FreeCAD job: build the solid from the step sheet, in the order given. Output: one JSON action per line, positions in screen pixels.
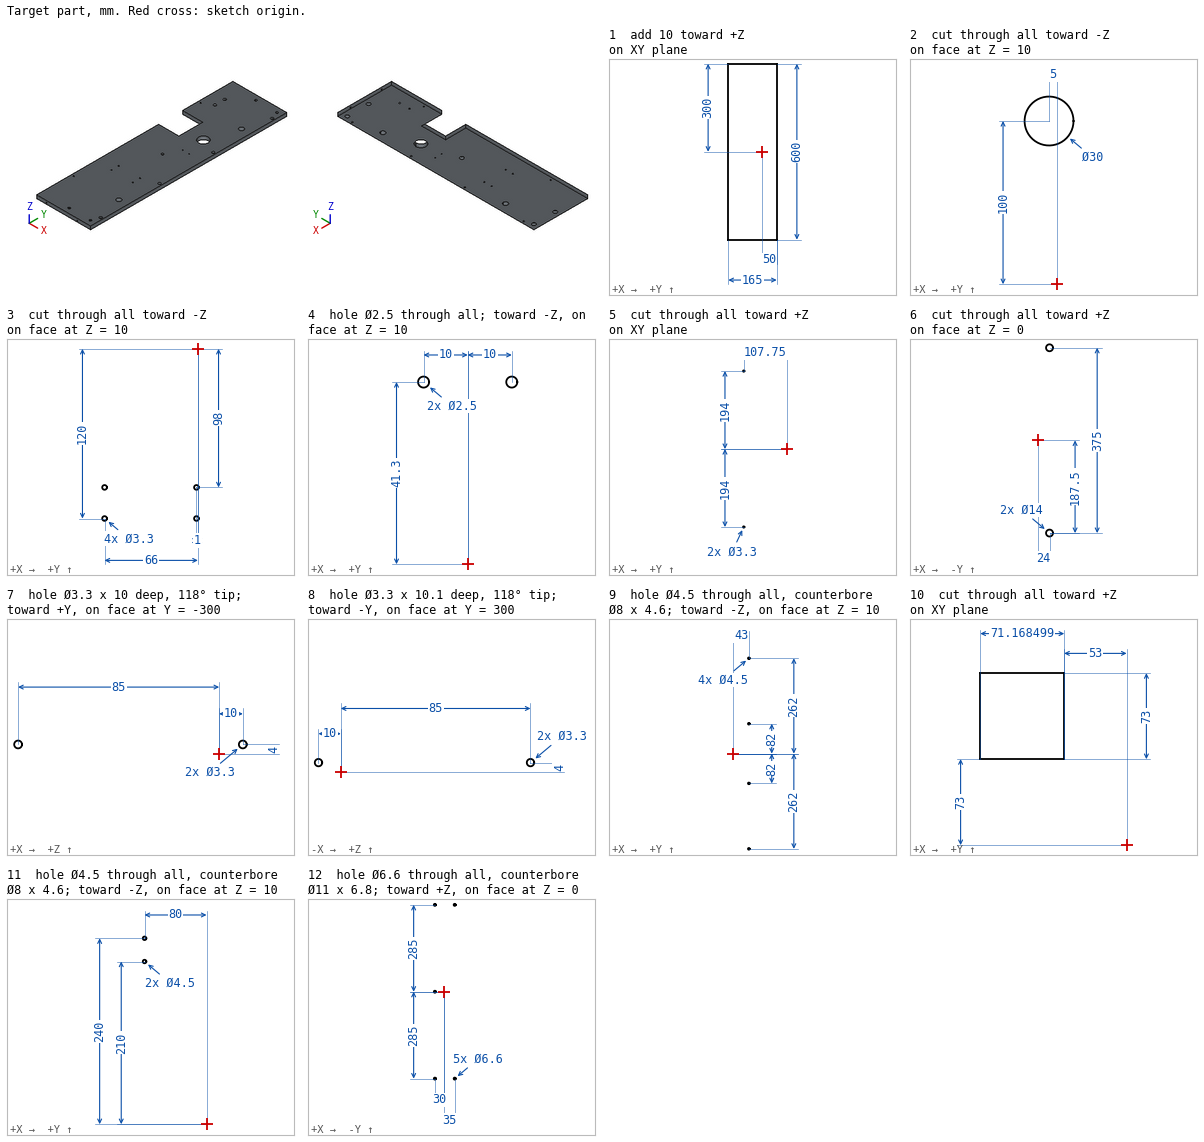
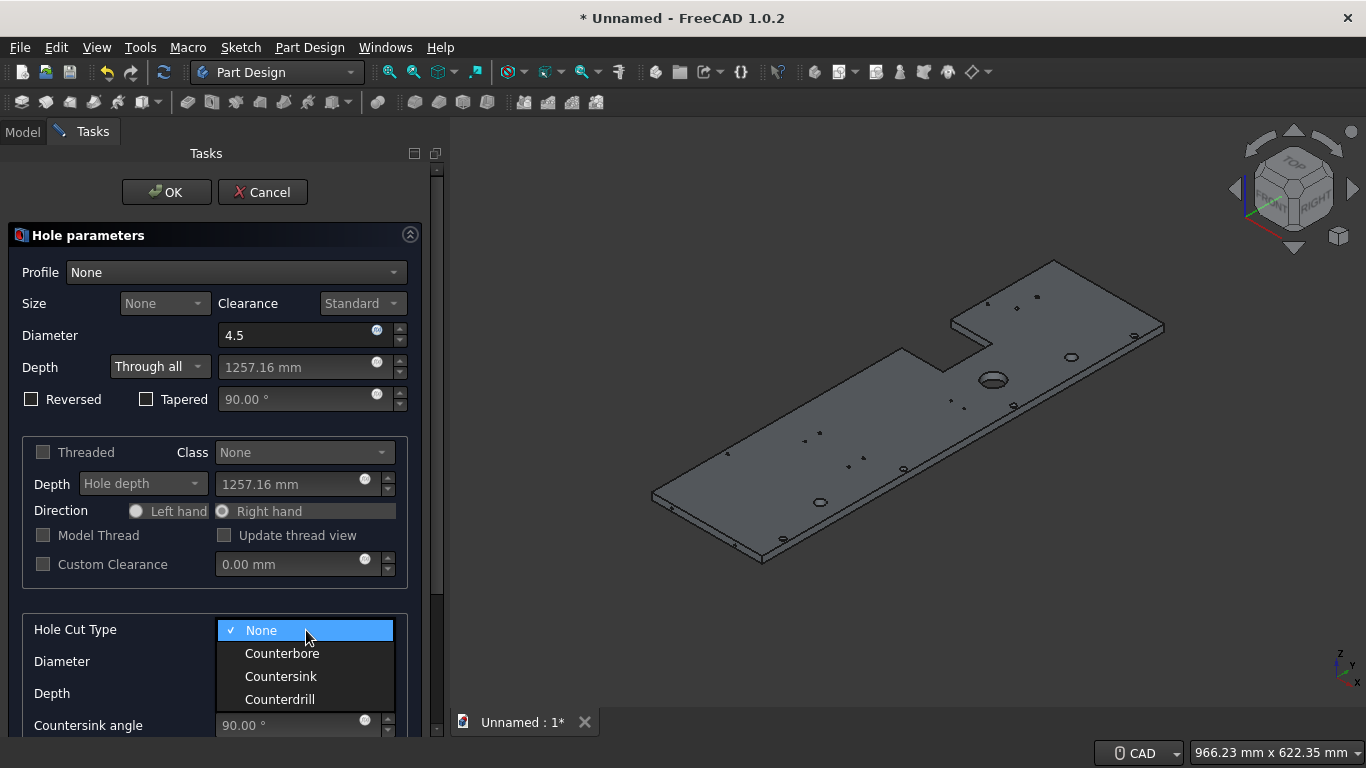
{"action": "left_click", "coordinate": [304, 654]}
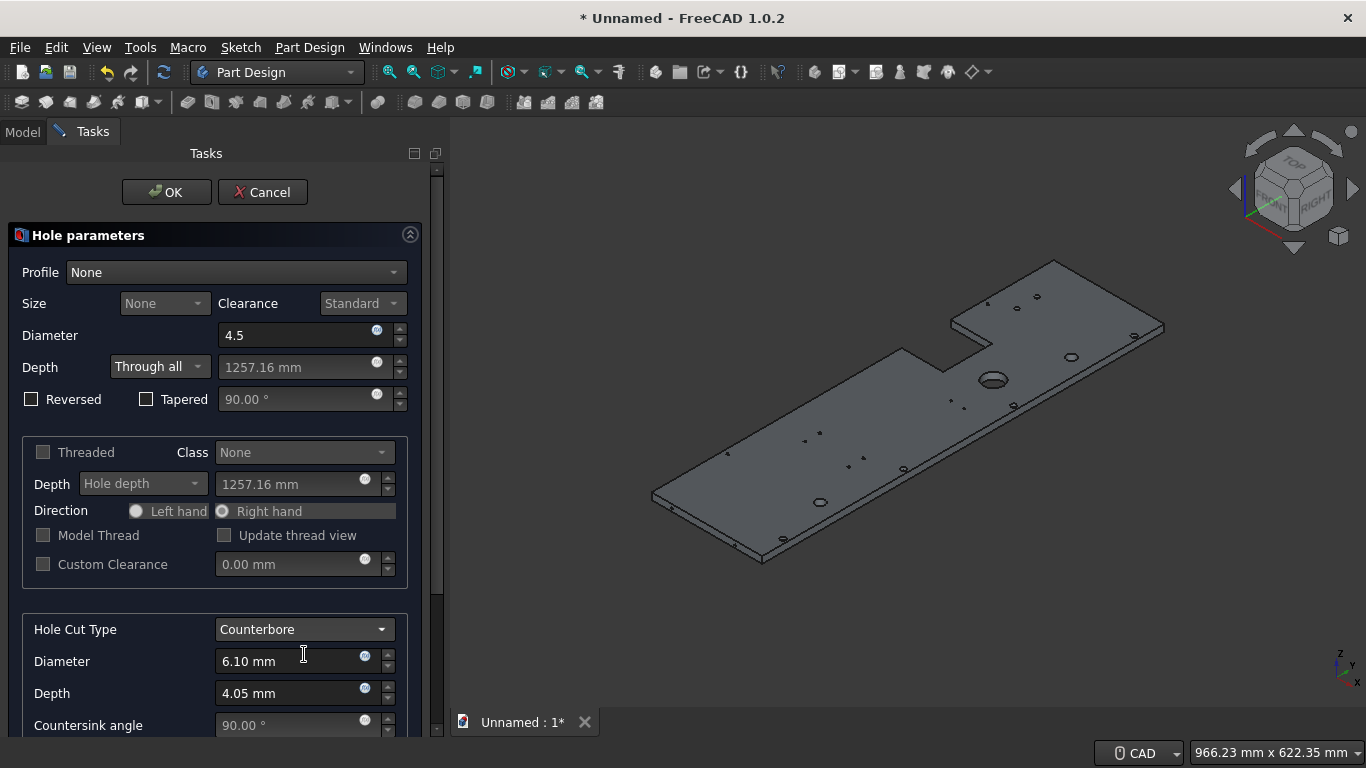
{"action": "triple_click", "coordinate": [298, 661]}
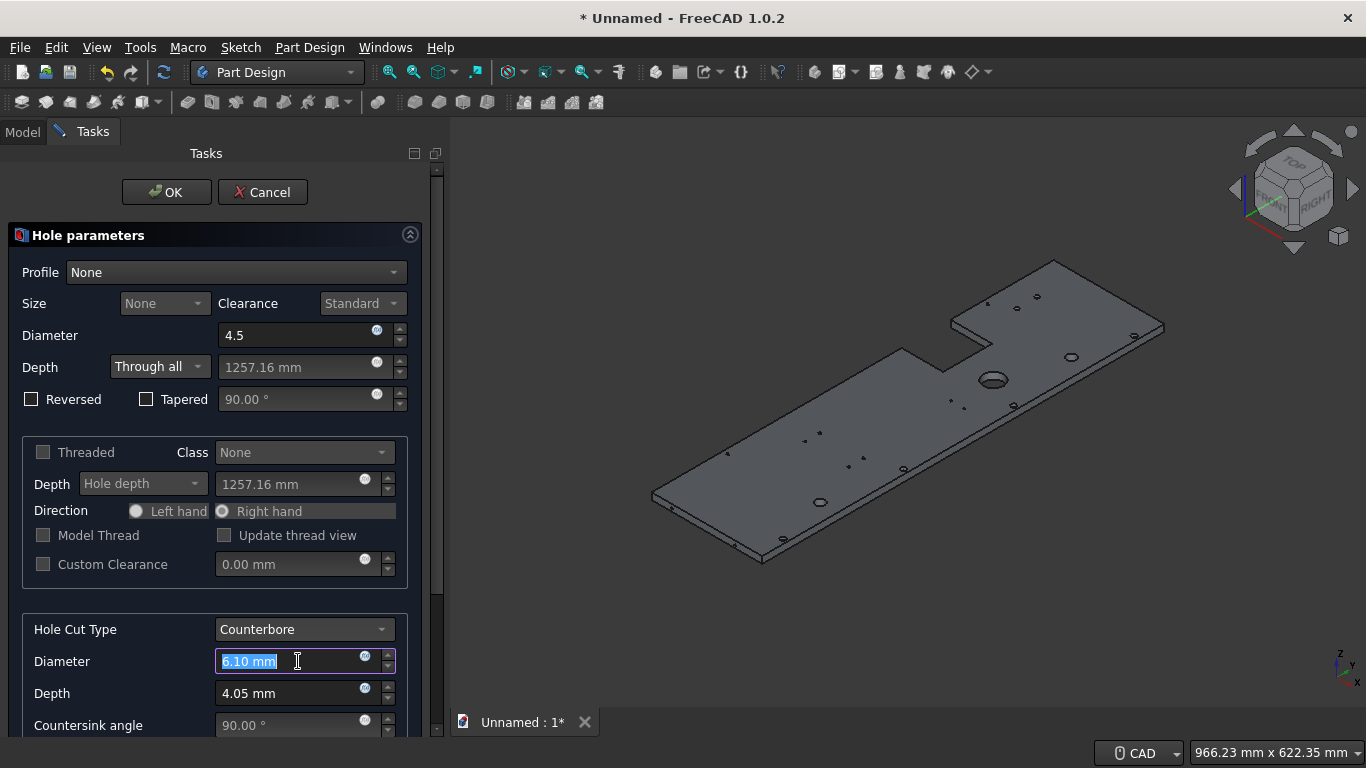
{"action": "type", "text": "8"}
{"action": "key", "text": "Tab"}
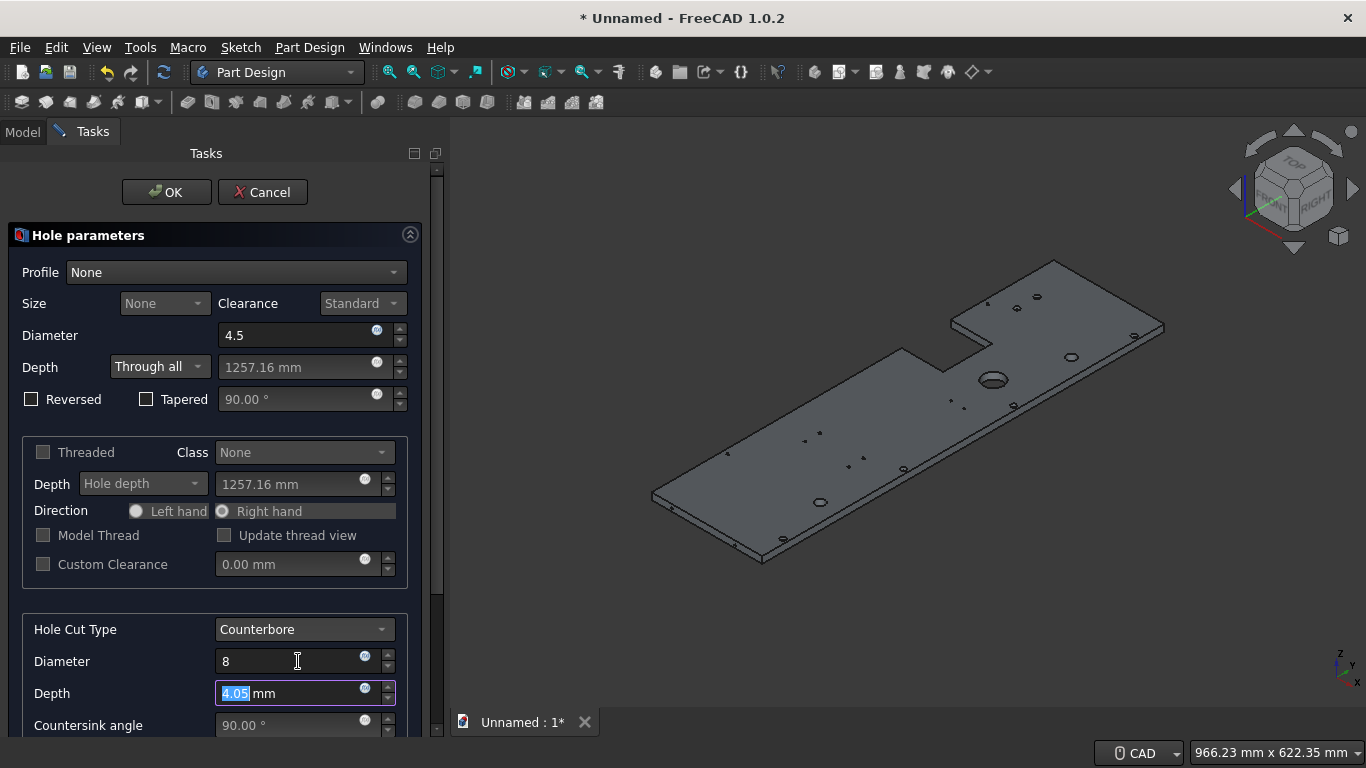
{"action": "type", "text": "4.6"}
{"action": "key", "text": "Tab"}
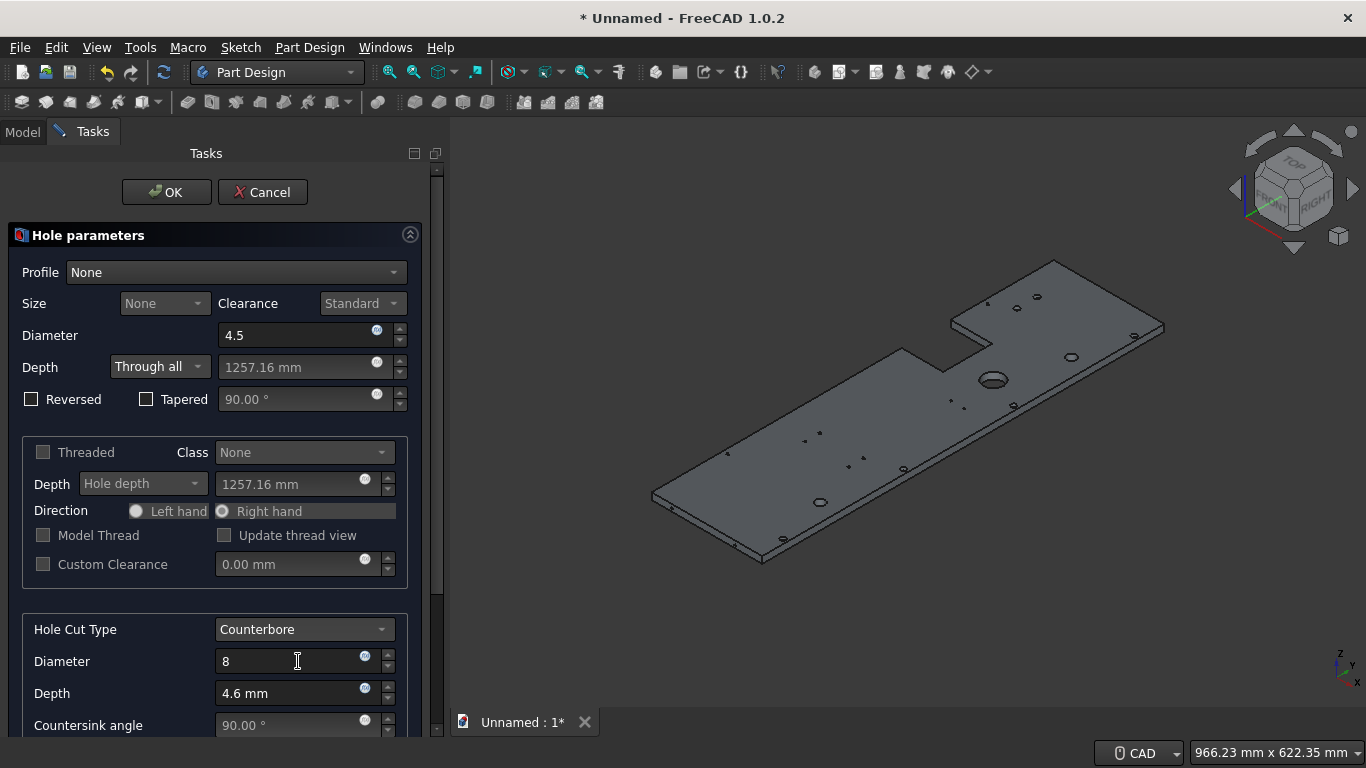
{"action": "left_click", "coordinate": [167, 192]}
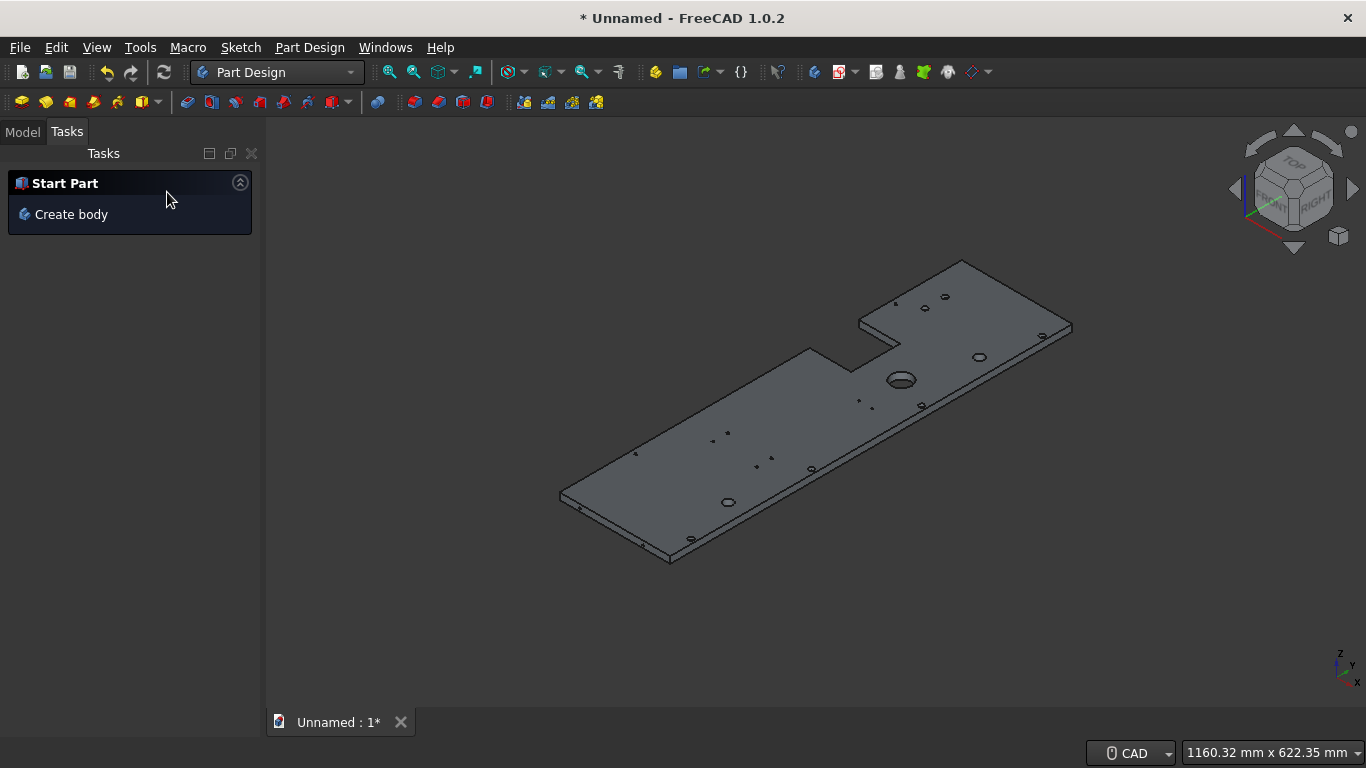
{"action": "key", "text": "5"}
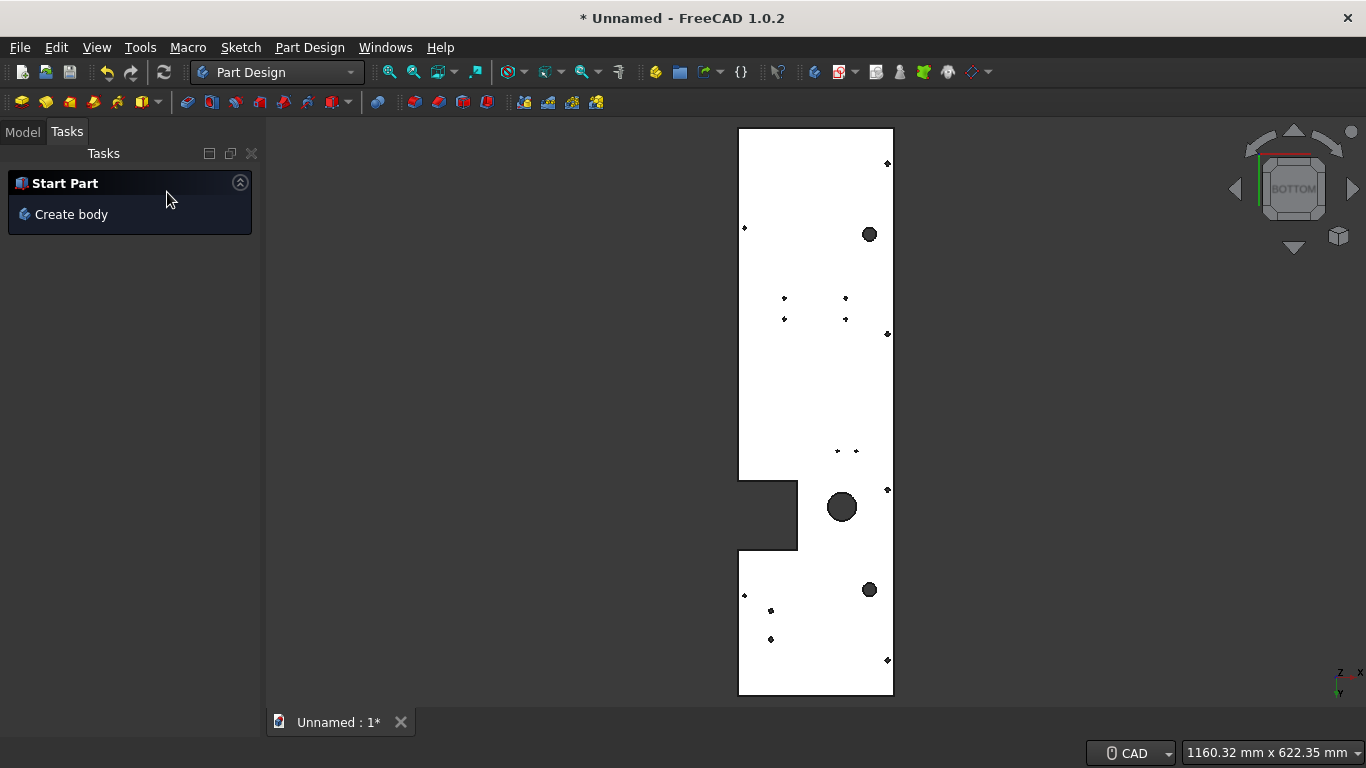
{"action": "left_click", "coordinate": [794, 411]}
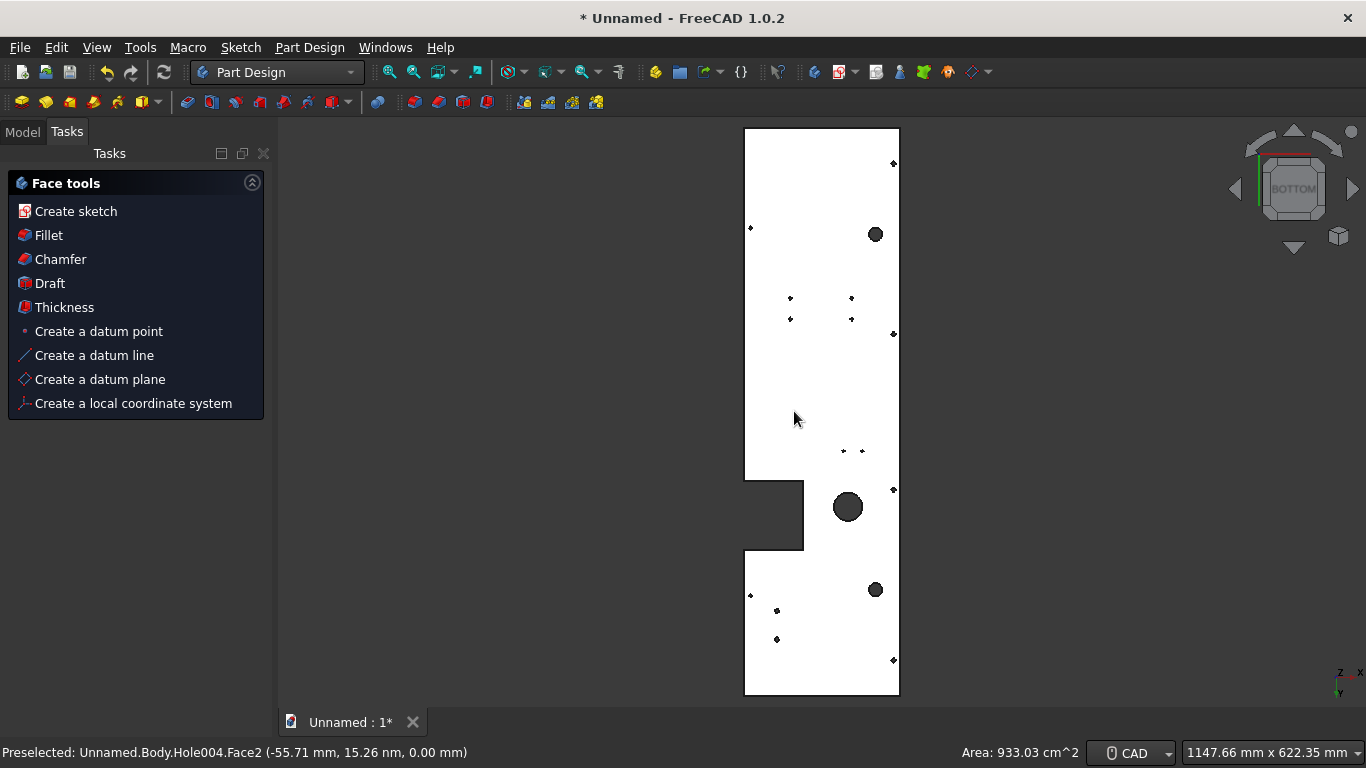
{"action": "left_click", "coordinate": [840, 72]}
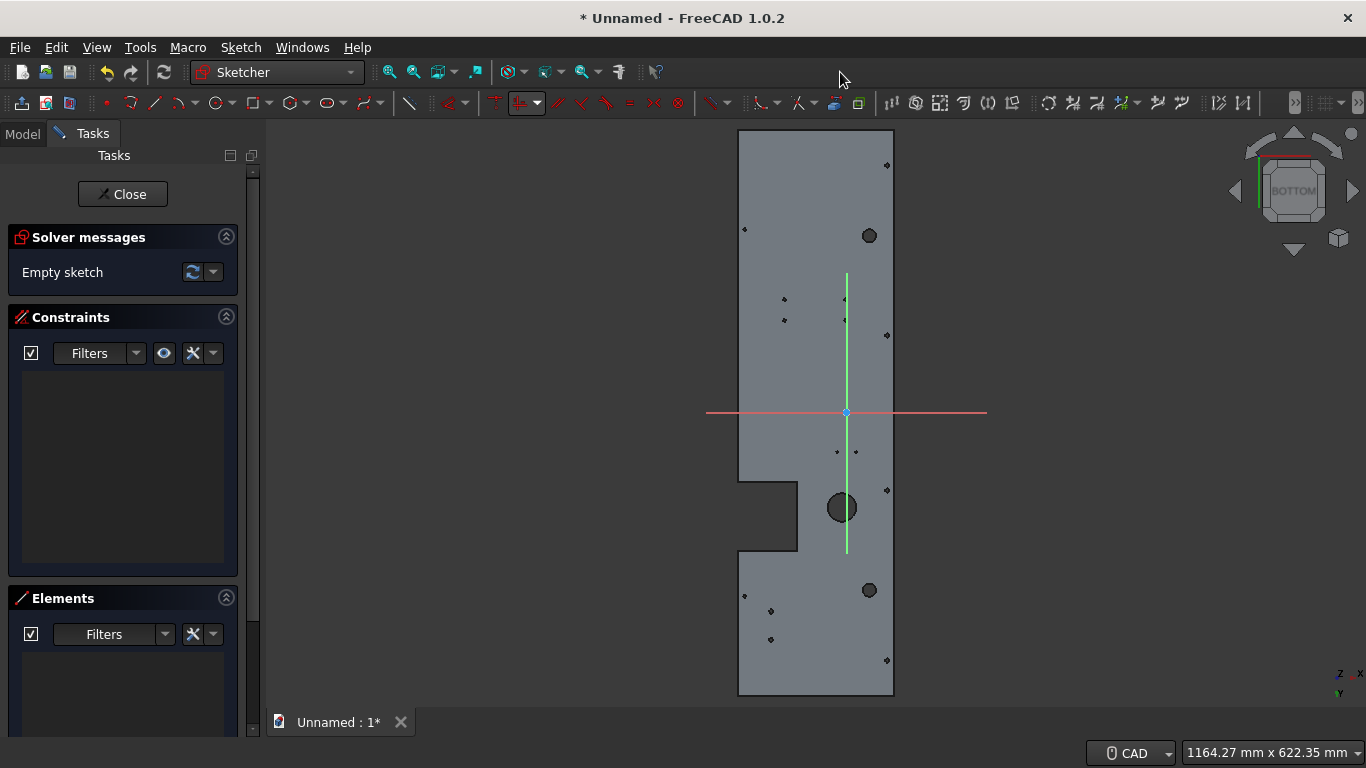
{"action": "scroll", "coordinate": [541, 413], "scroll_direction": "down", "scroll_amount": 2}